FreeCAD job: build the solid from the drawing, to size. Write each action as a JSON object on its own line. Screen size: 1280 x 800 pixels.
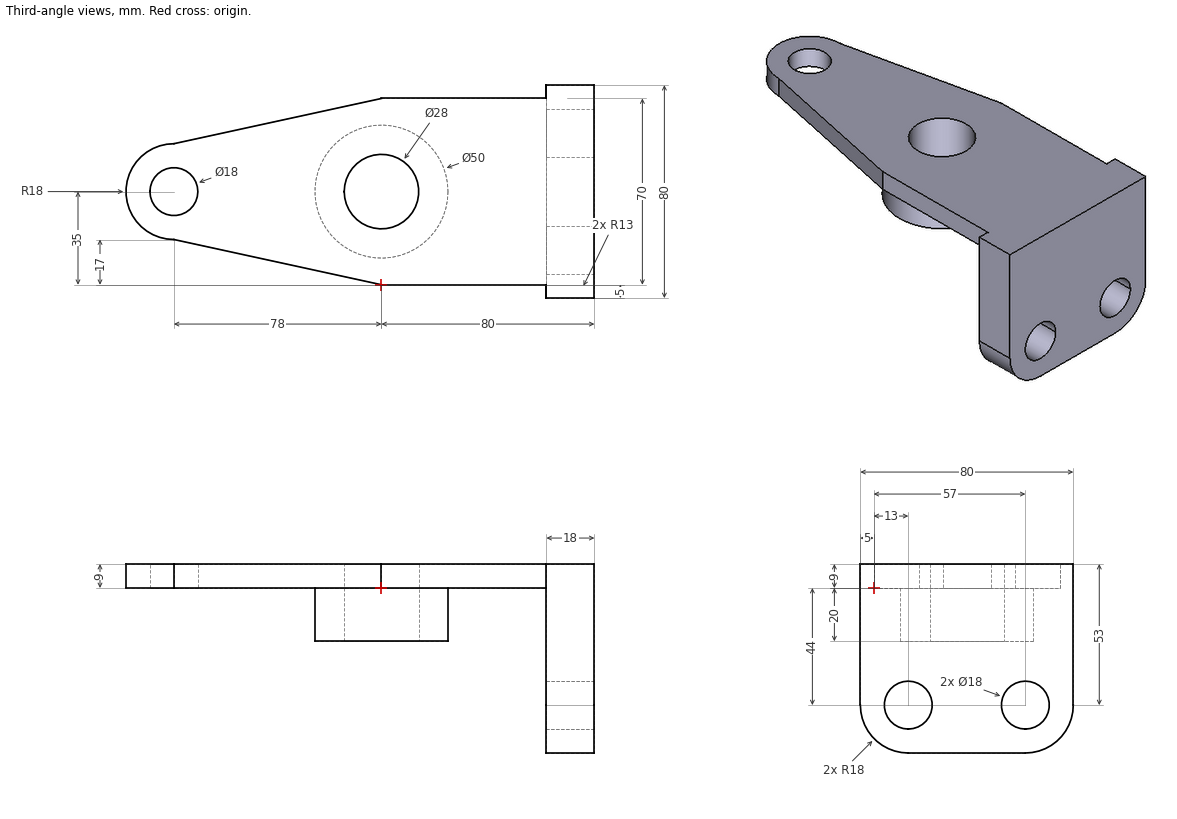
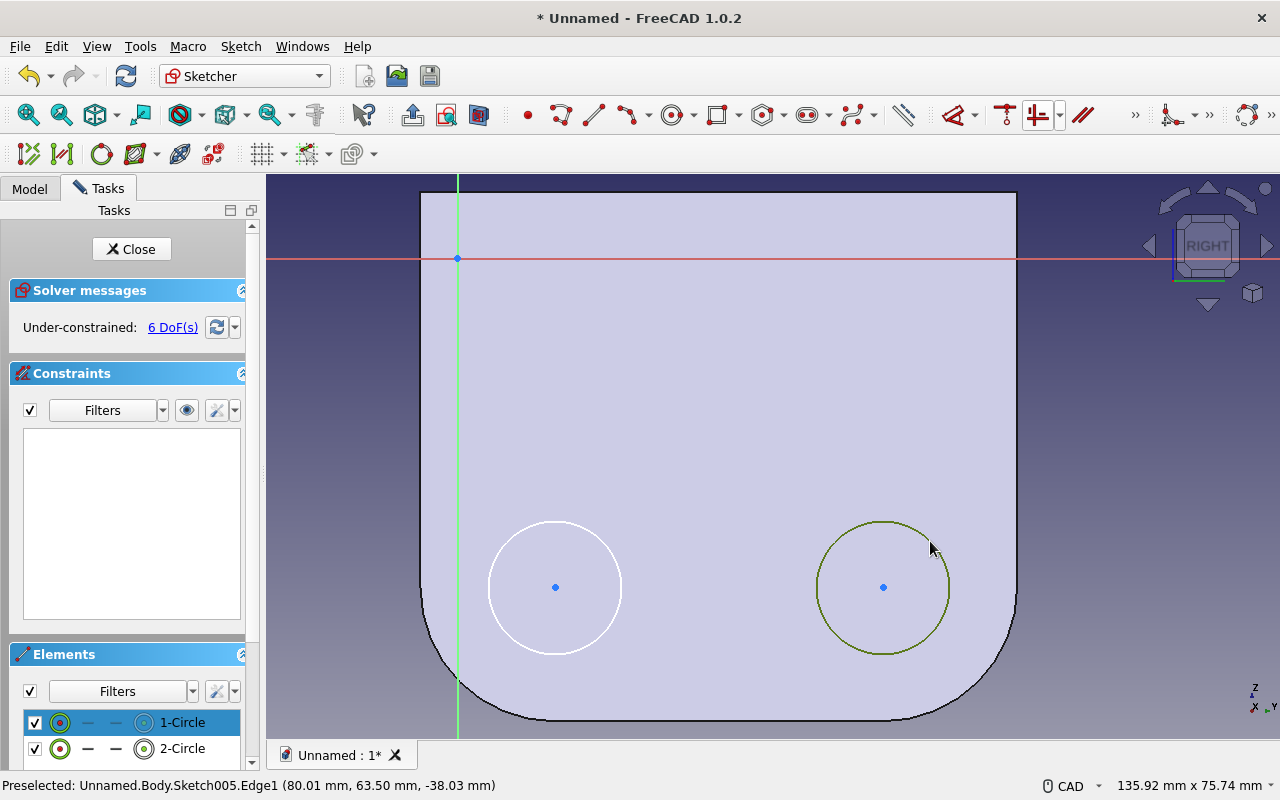
{"action": "left_click", "coordinate": [602, 541]}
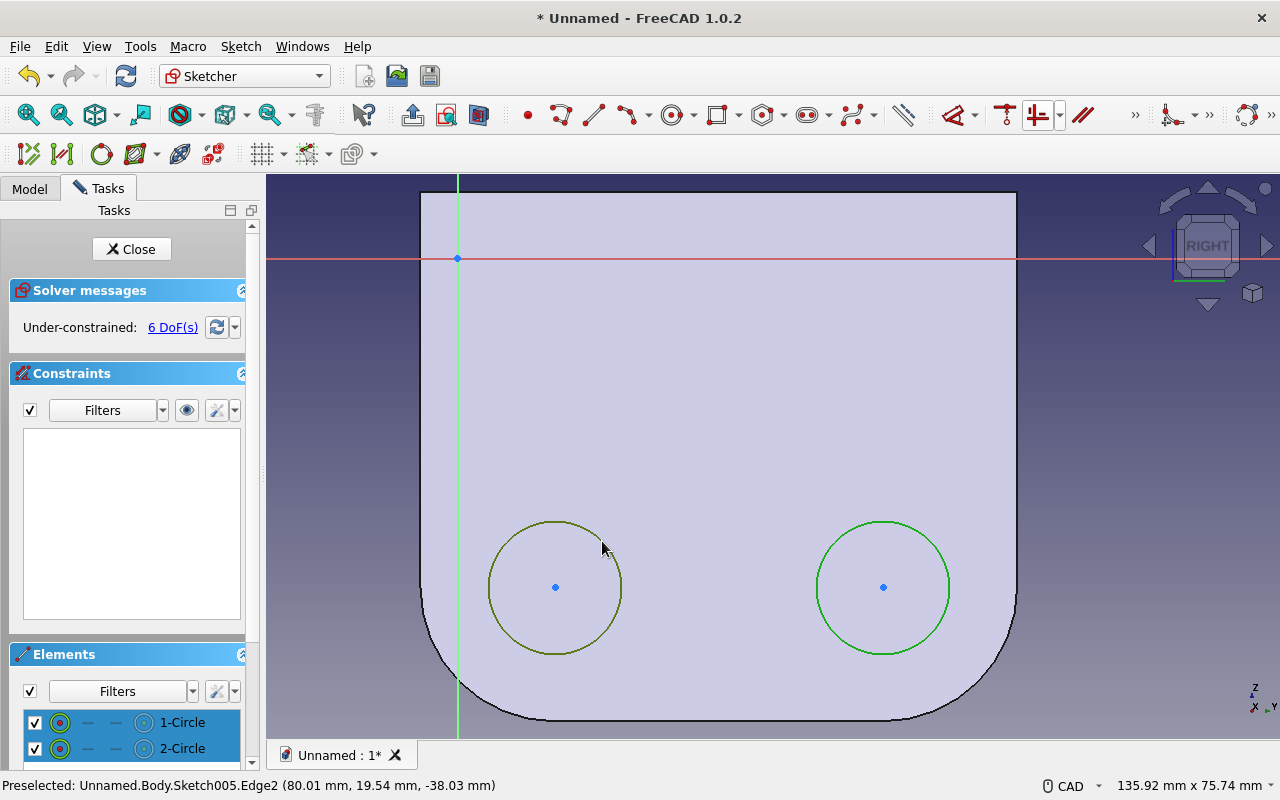
{"action": "key", "text": "e"}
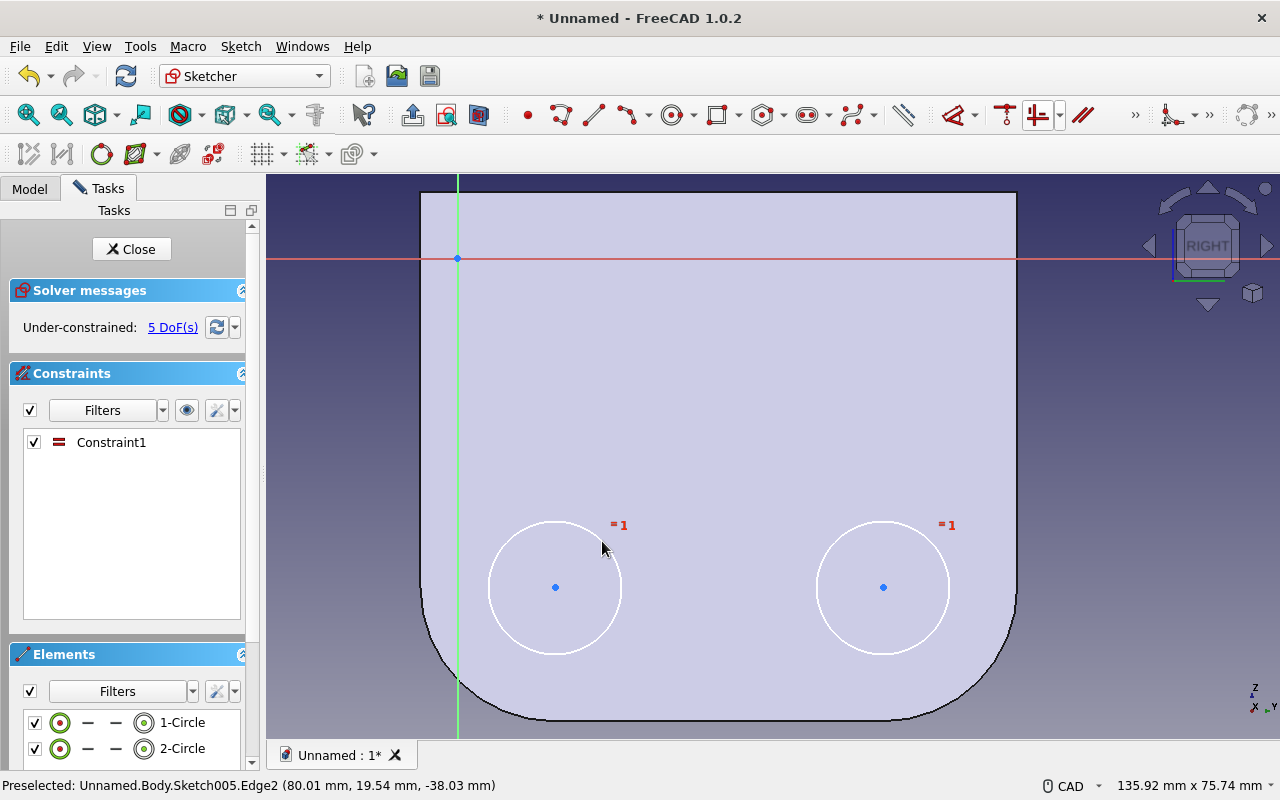
{"action": "left_click", "coordinate": [883, 588]}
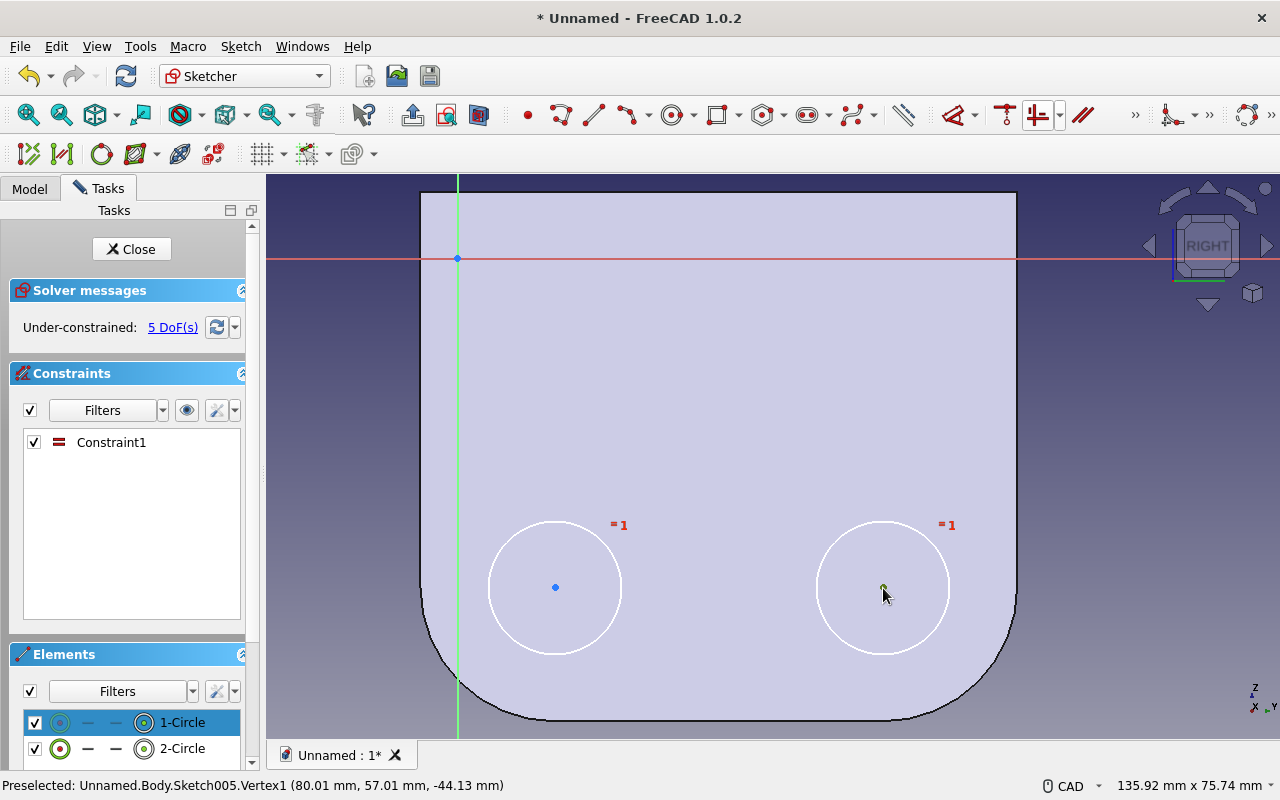
{"action": "left_click", "coordinate": [555, 588]}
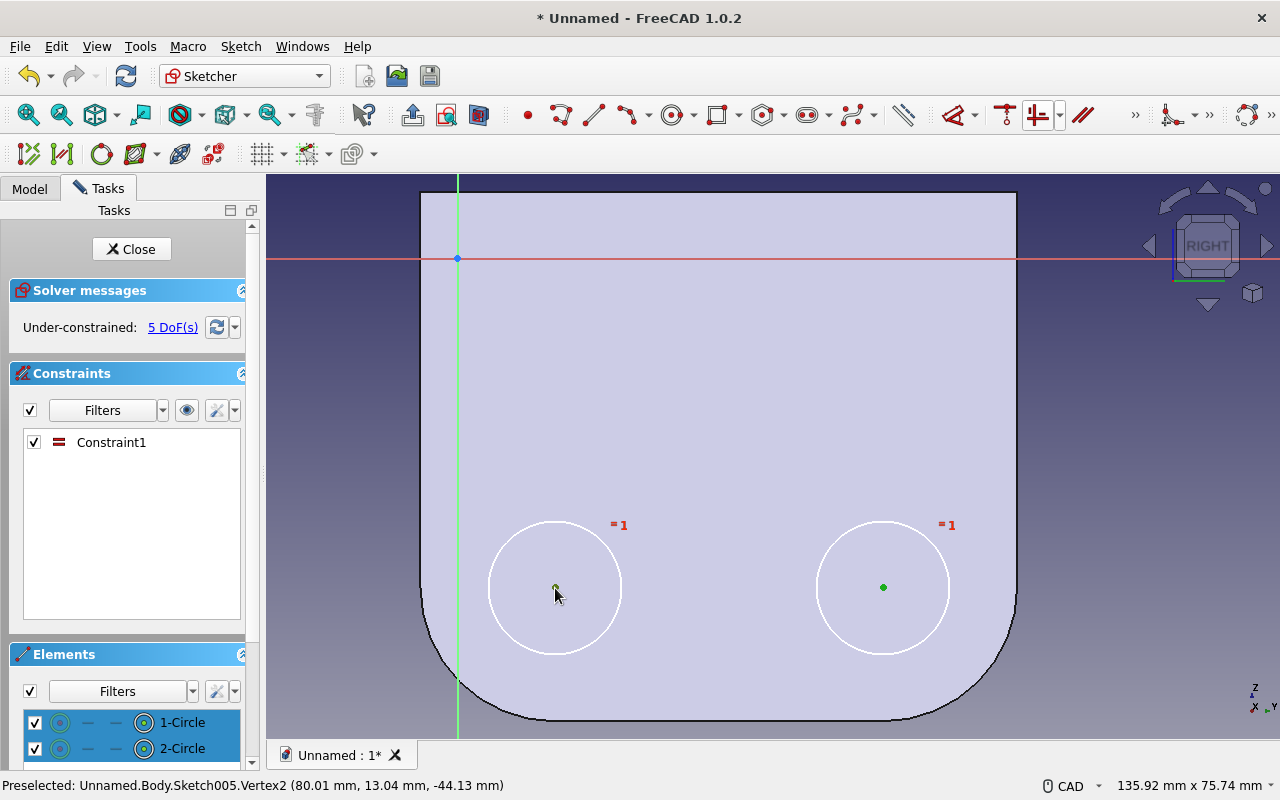
{"action": "key", "text": "h"}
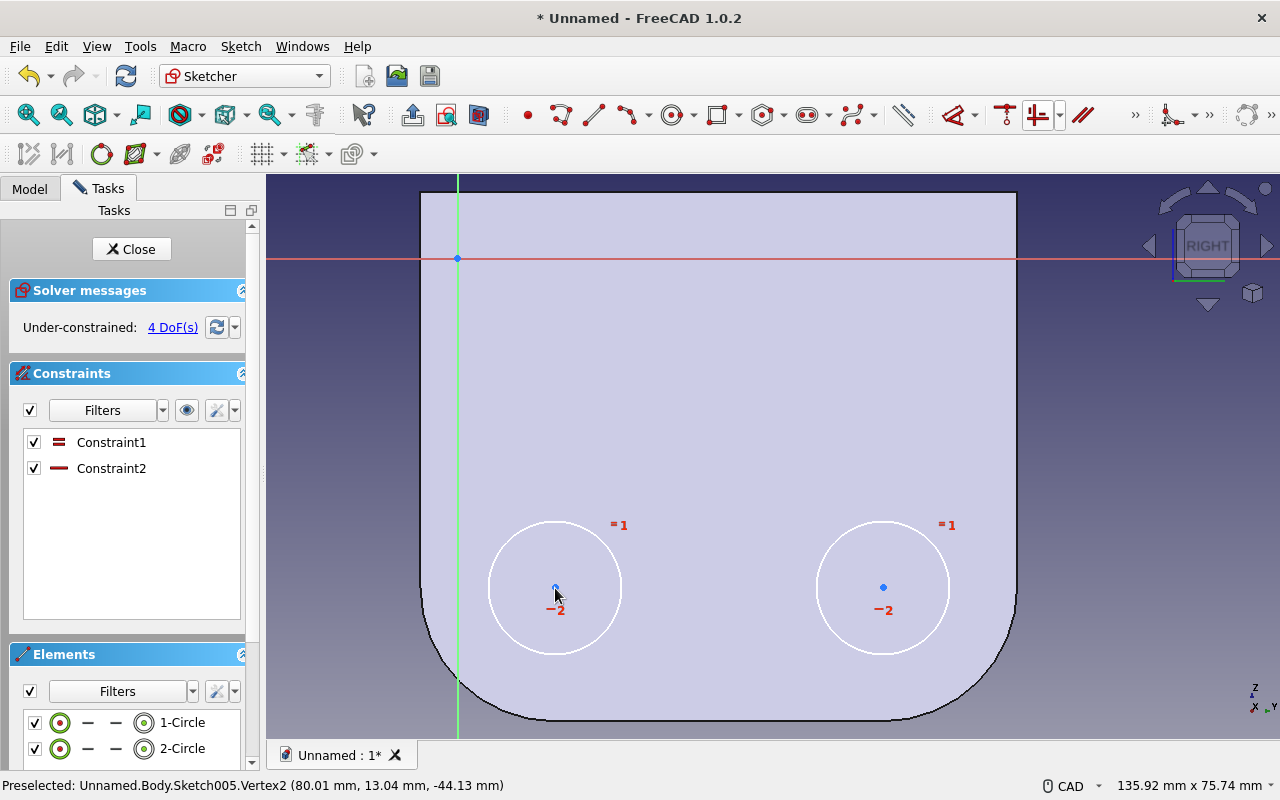
{"action": "left_click", "coordinate": [952, 116]}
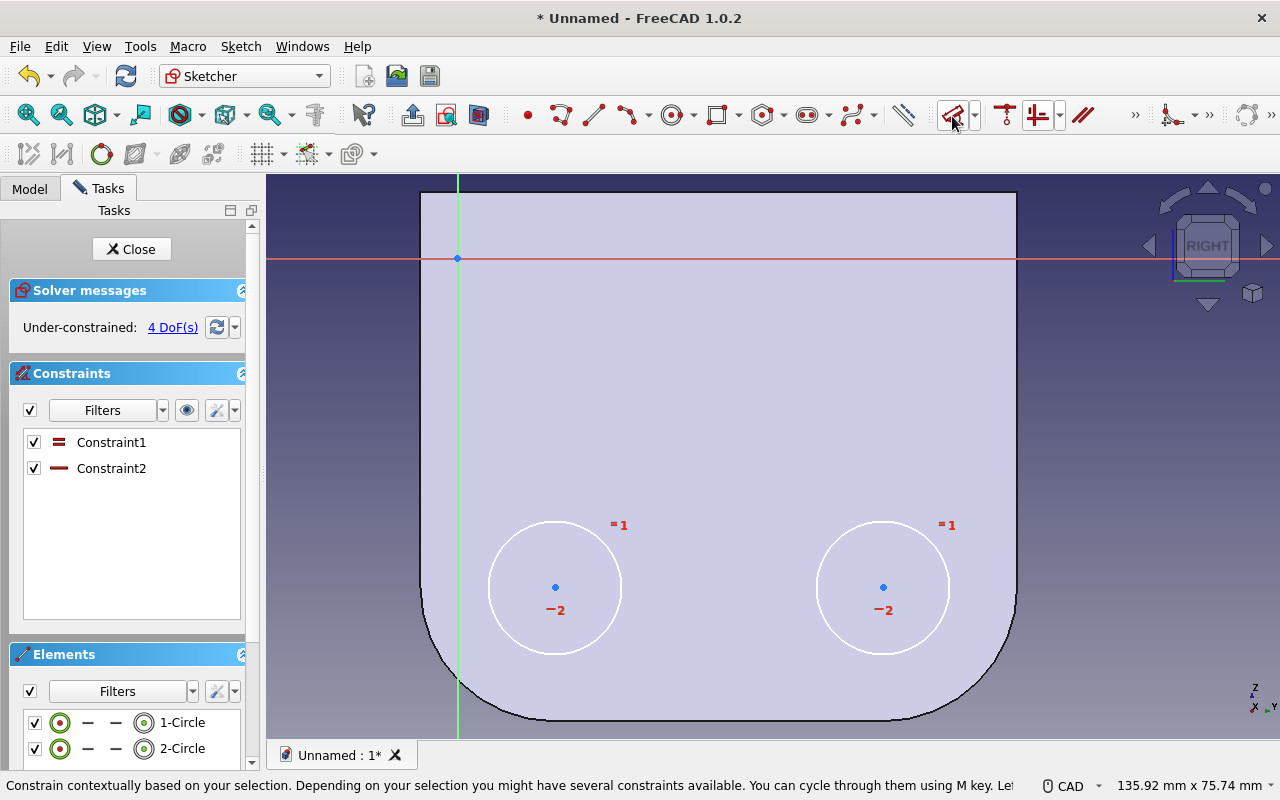
{"action": "left_click", "coordinate": [930, 541]}
{"action": "left_click", "coordinate": [953, 518]}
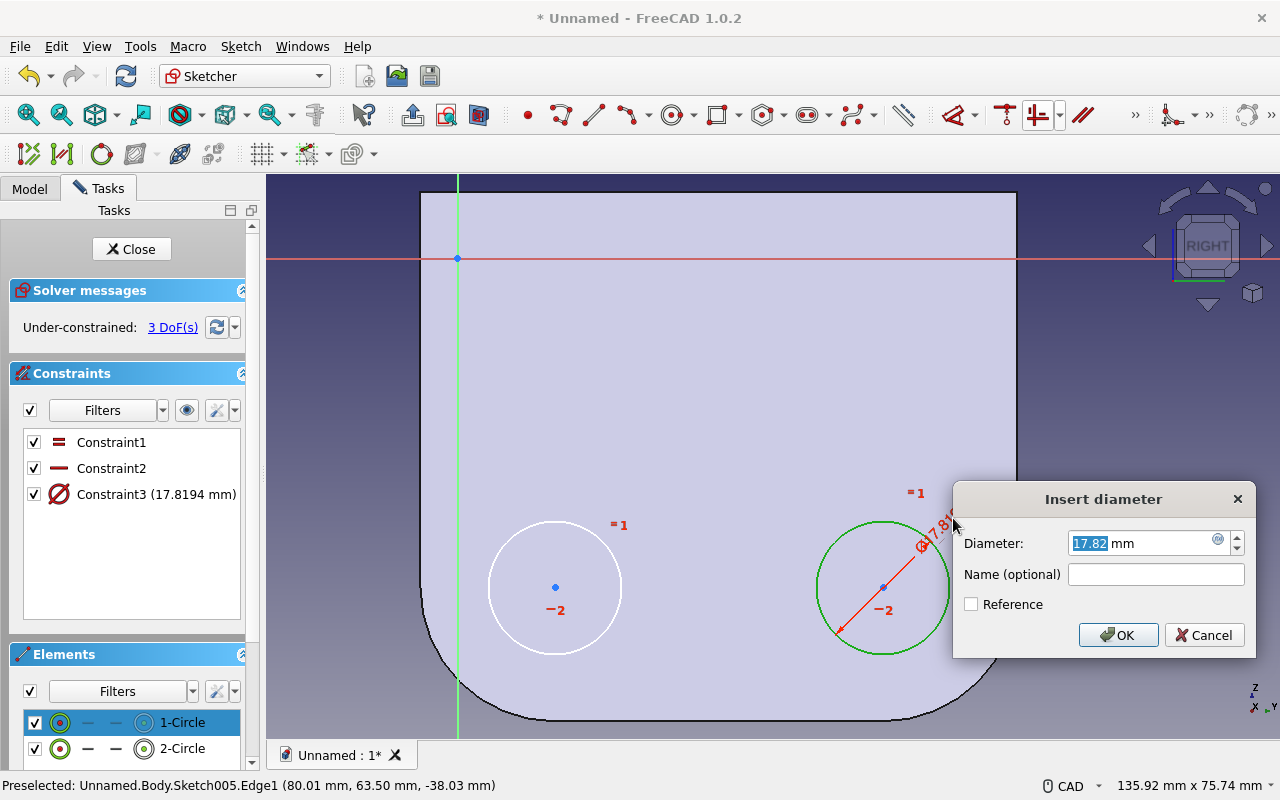
{"action": "type", "text": "18"}
{"action": "key", "text": "Return"}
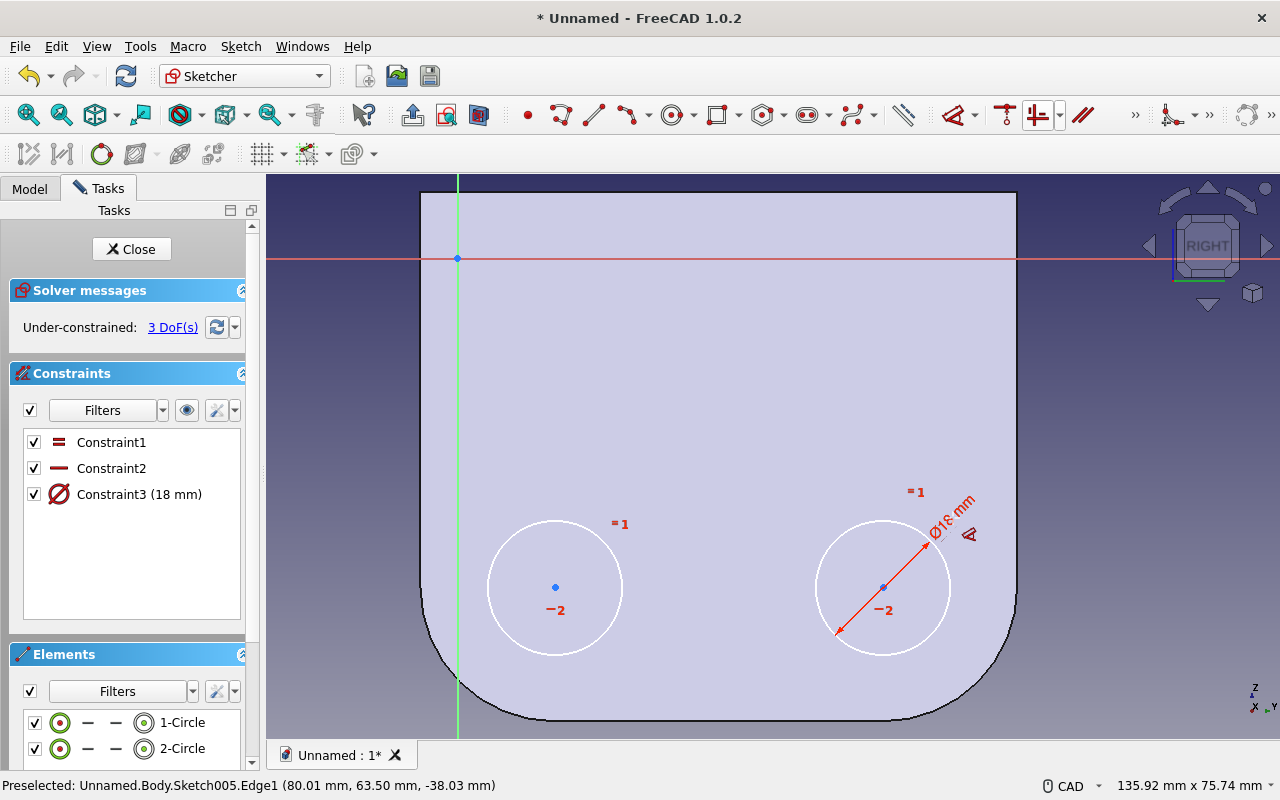
{"action": "left_click", "coordinate": [883, 588]}
{"action": "left_click", "coordinate": [670, 225]}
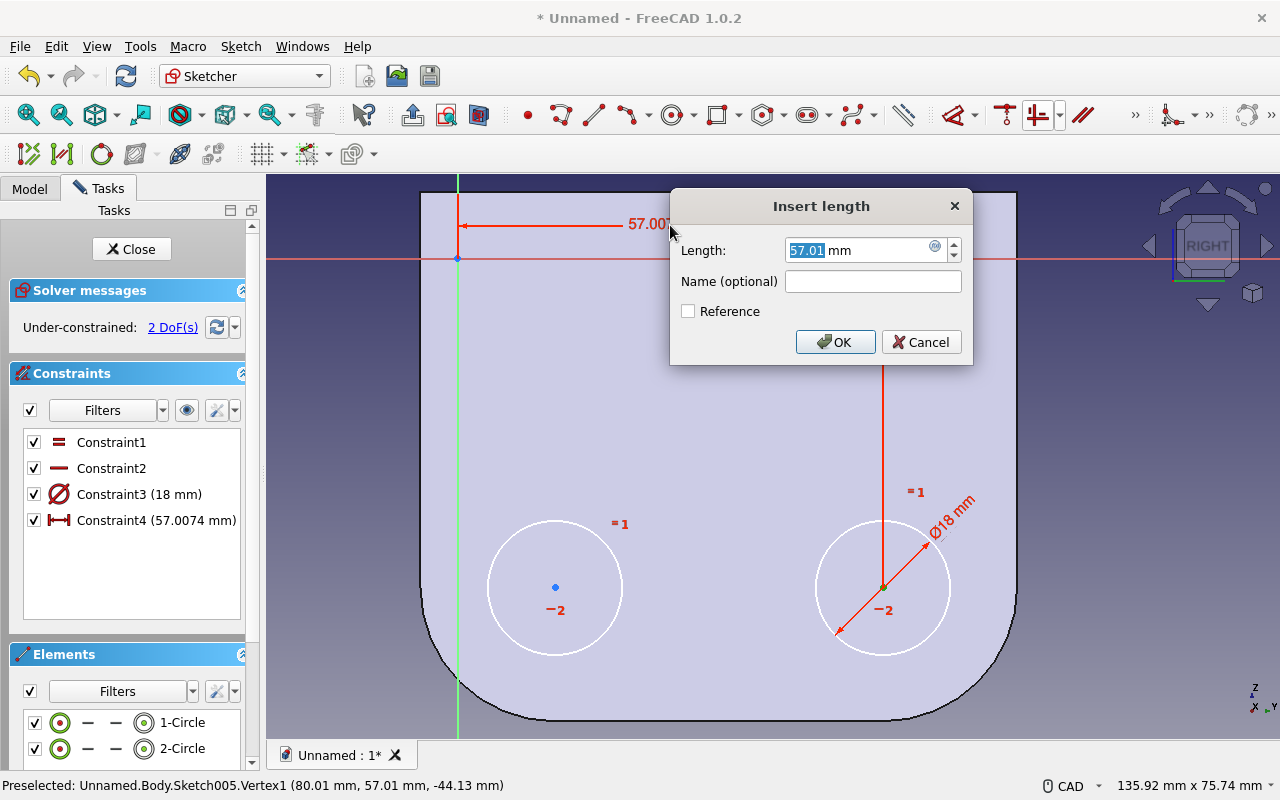
{"action": "type", "text": "57"}
{"action": "key", "text": "Return"}